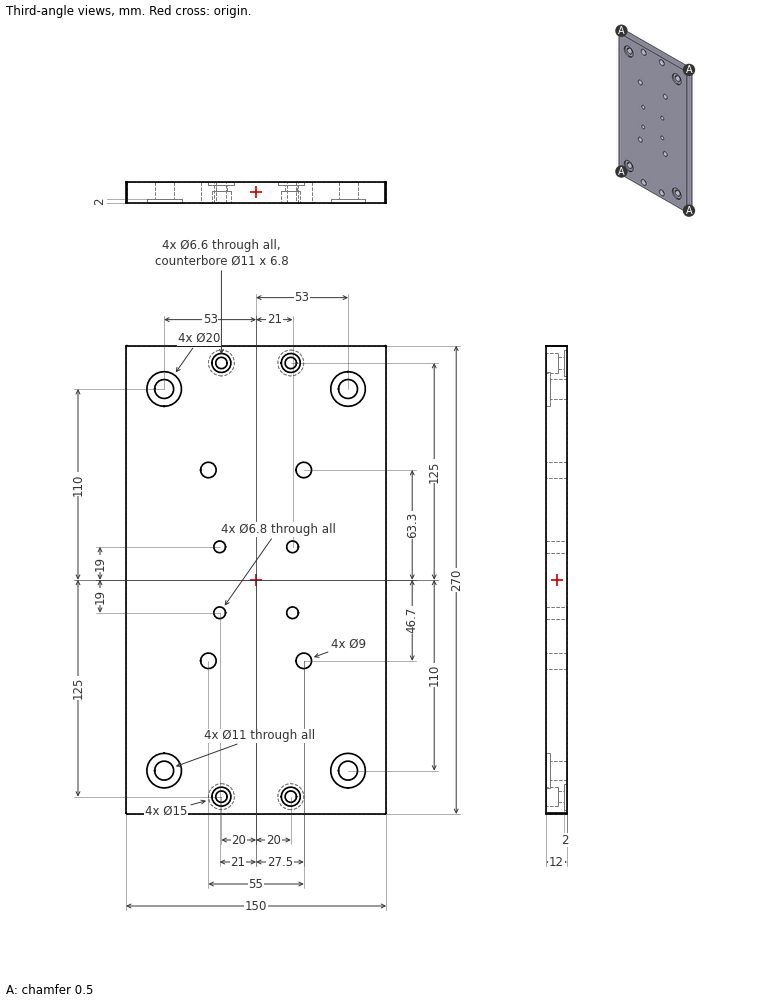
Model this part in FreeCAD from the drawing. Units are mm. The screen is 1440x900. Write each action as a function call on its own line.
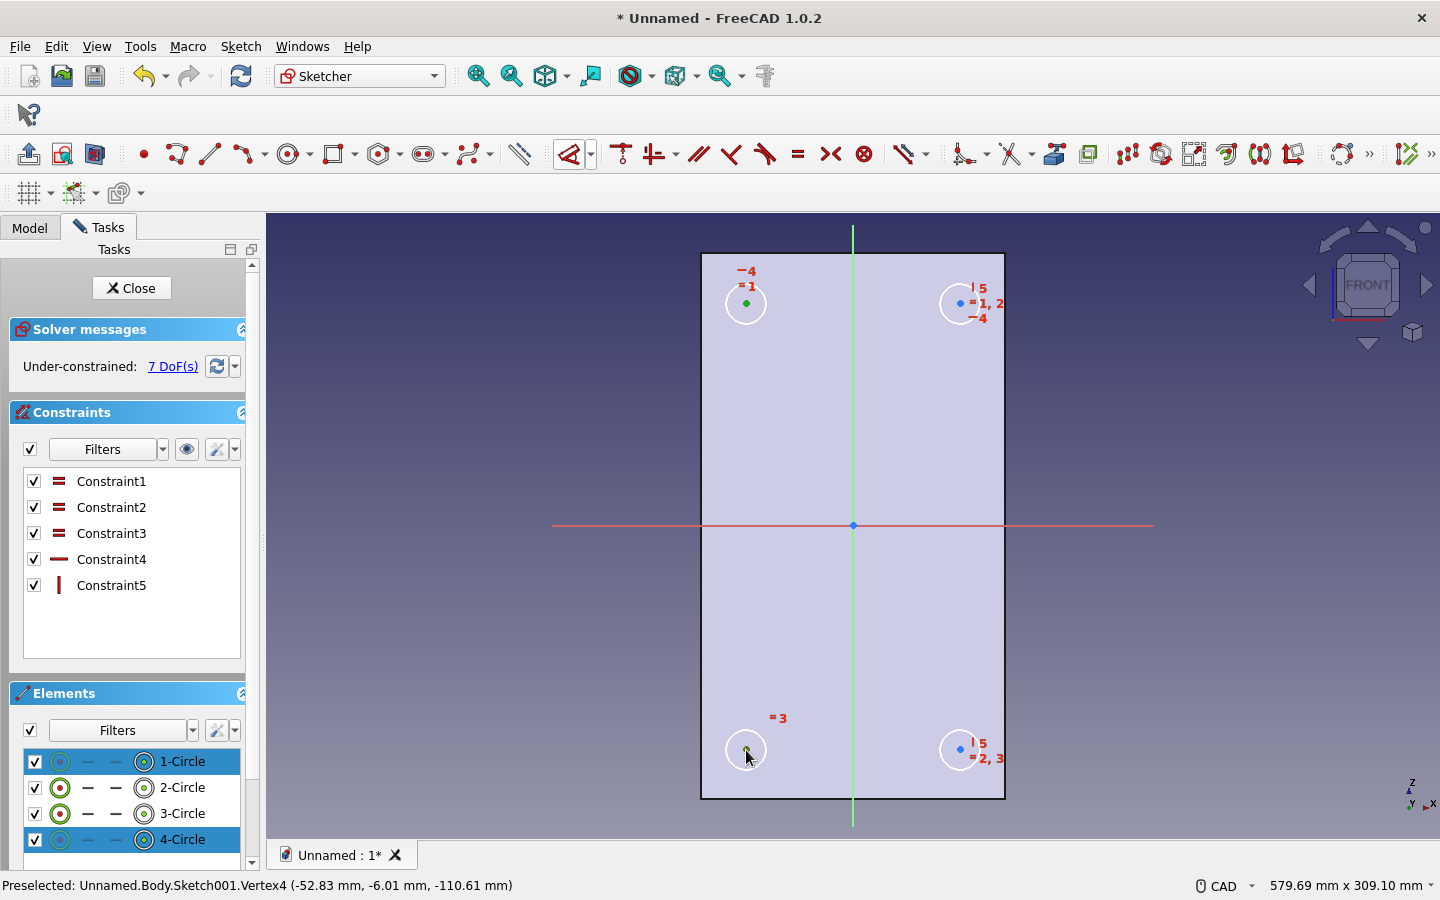
key(v)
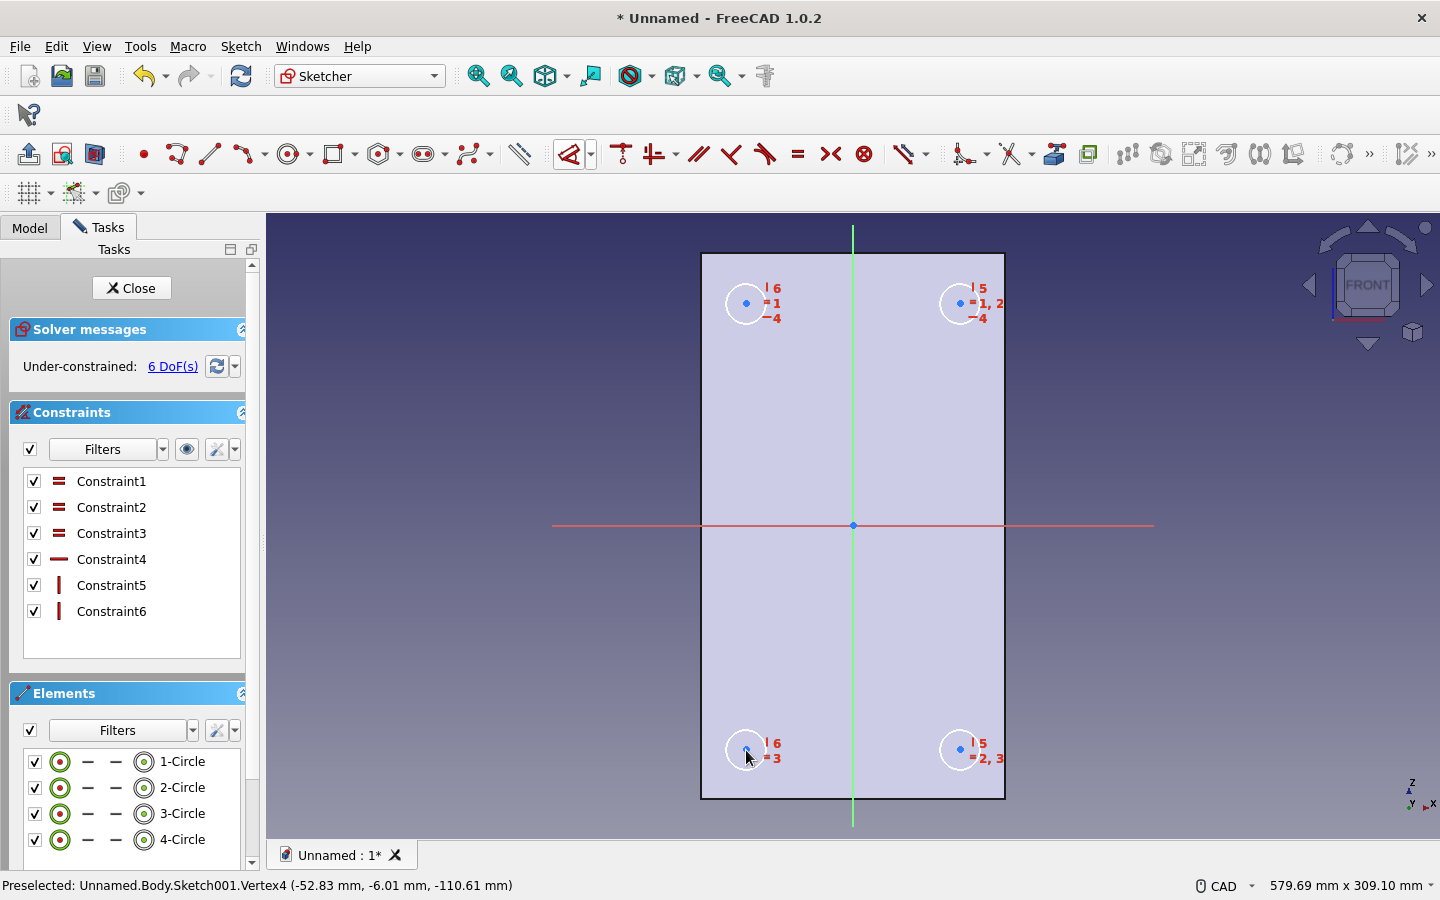
click(960, 750)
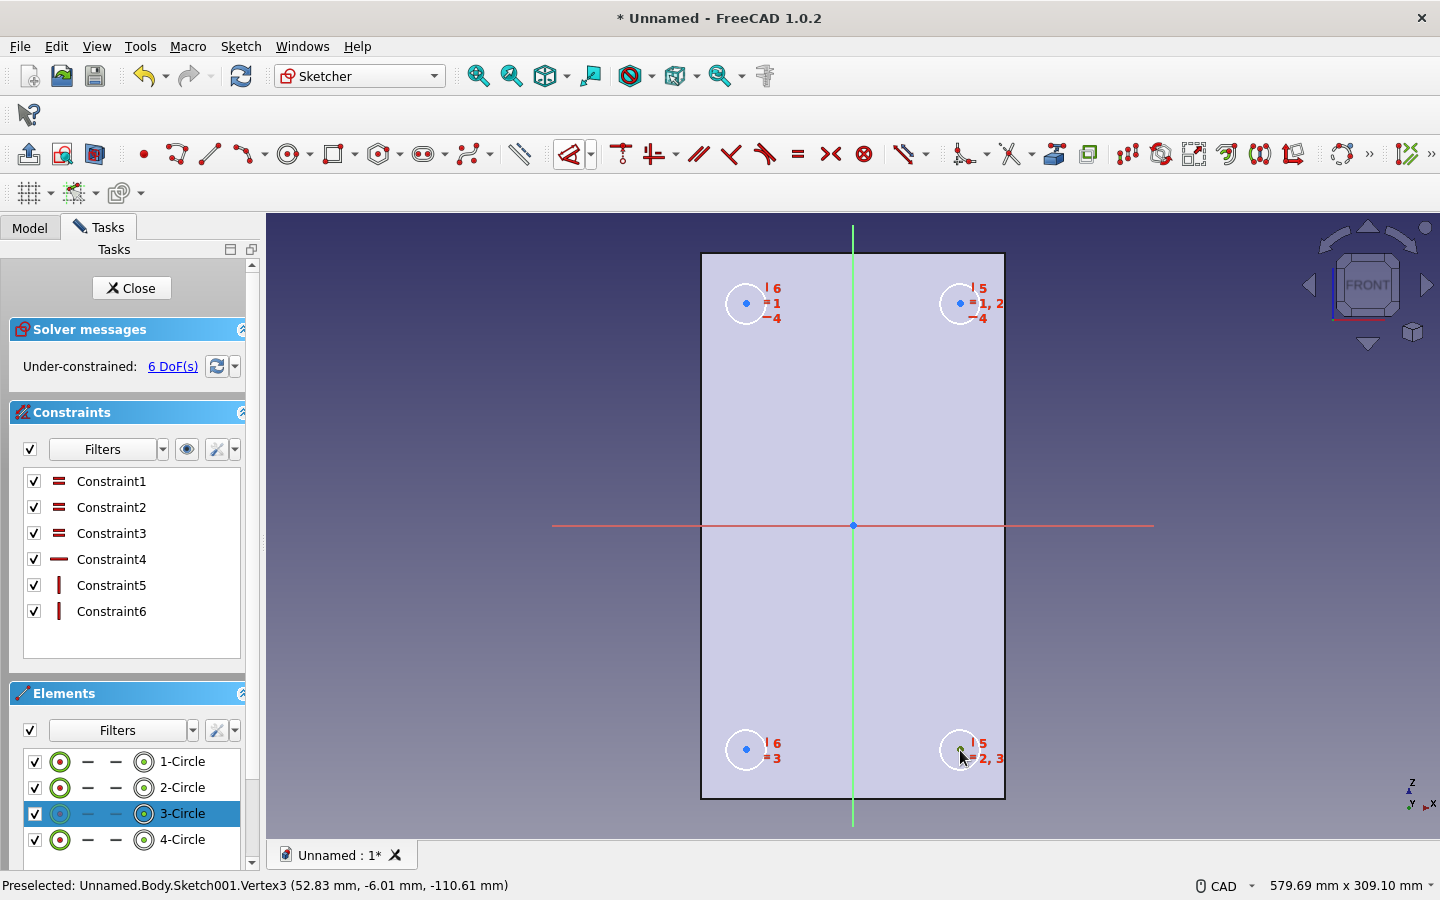
click(746, 750)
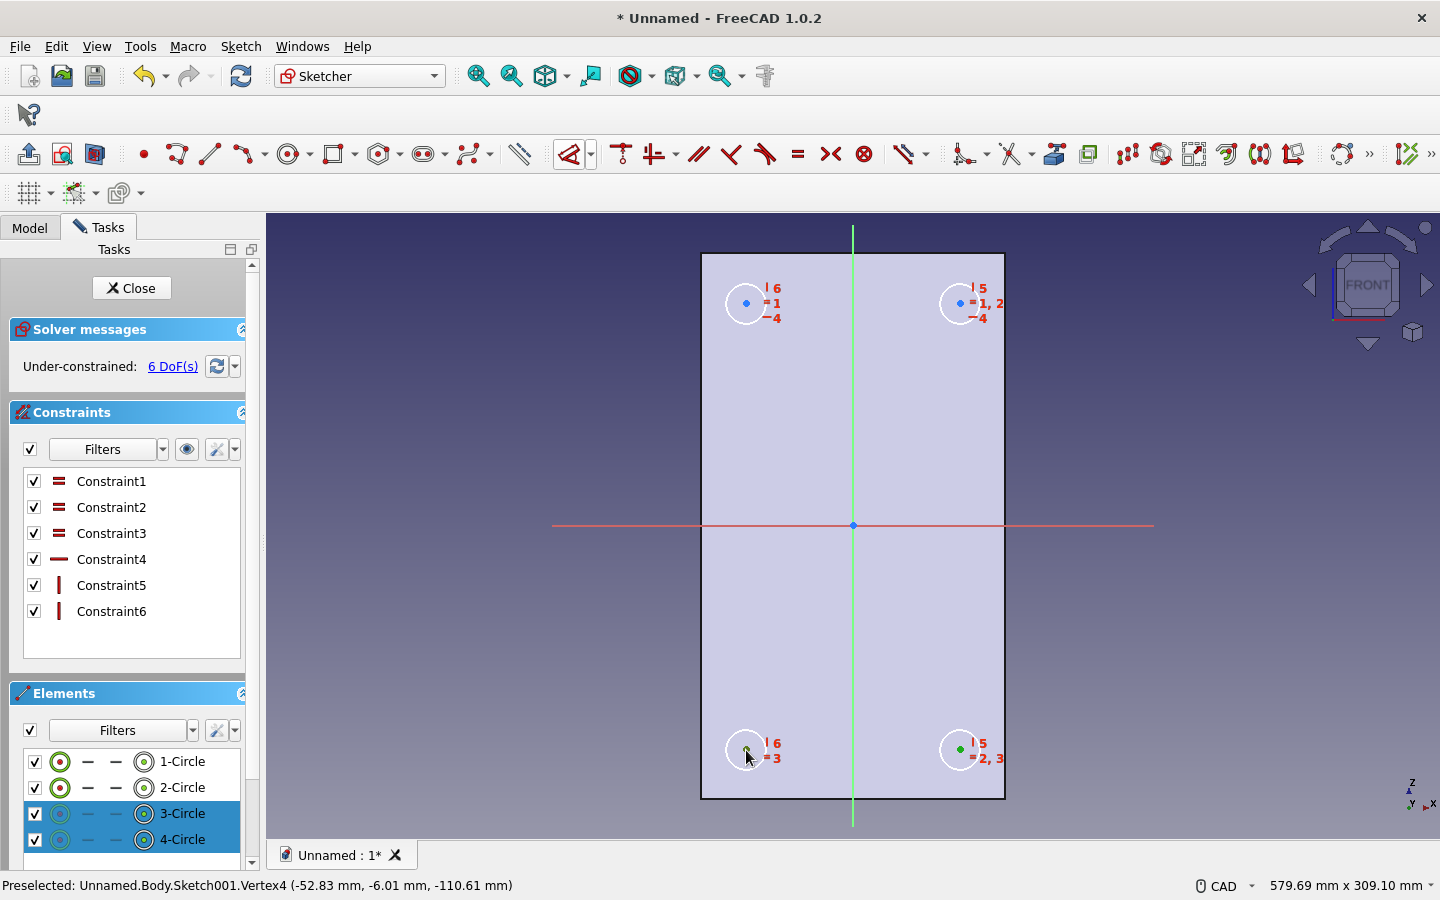
key(h)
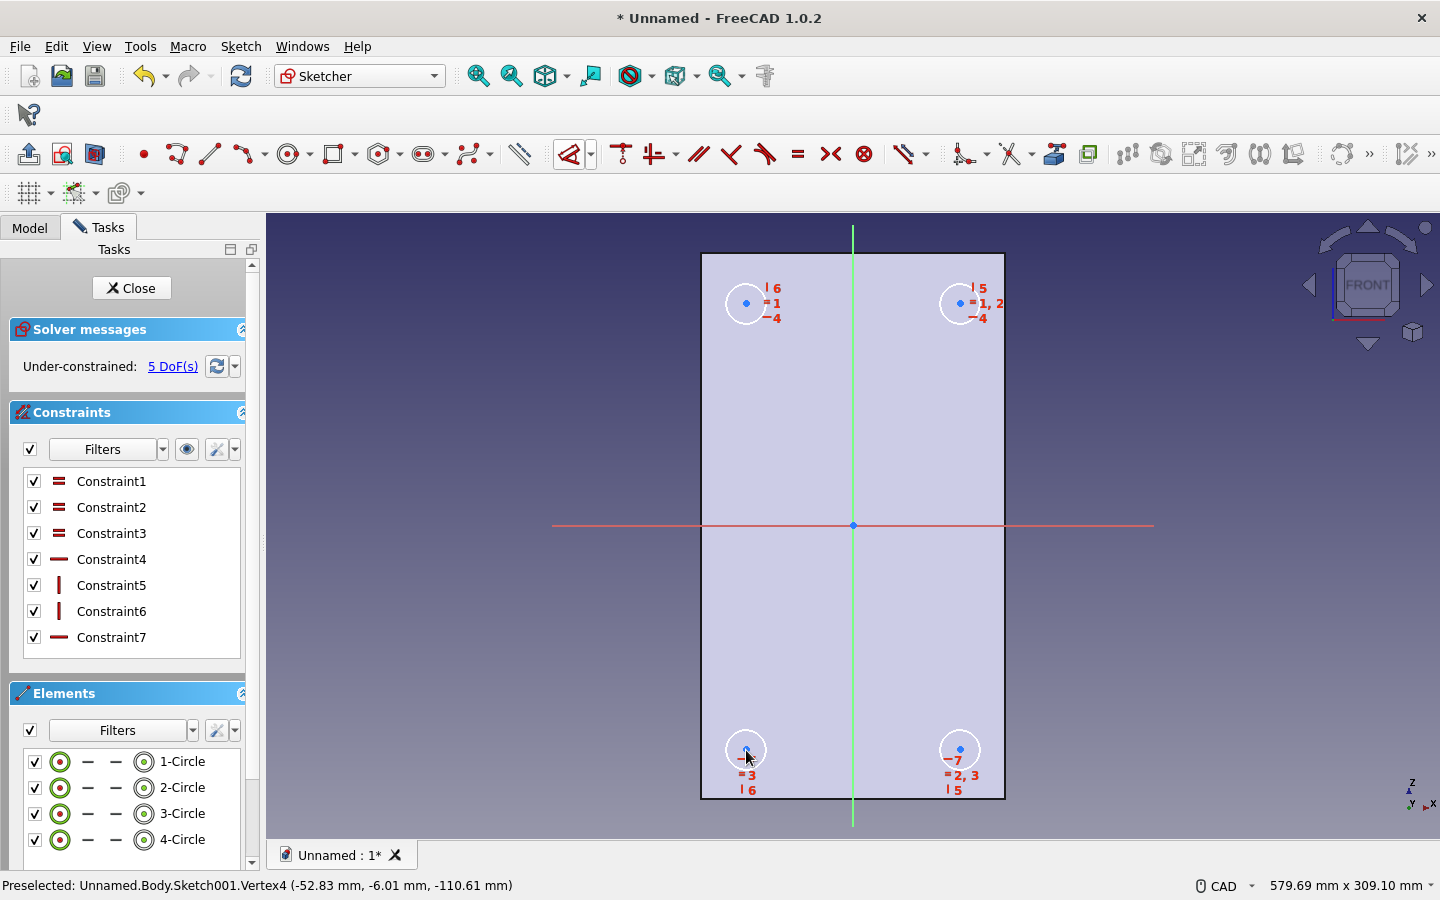
click(760, 290)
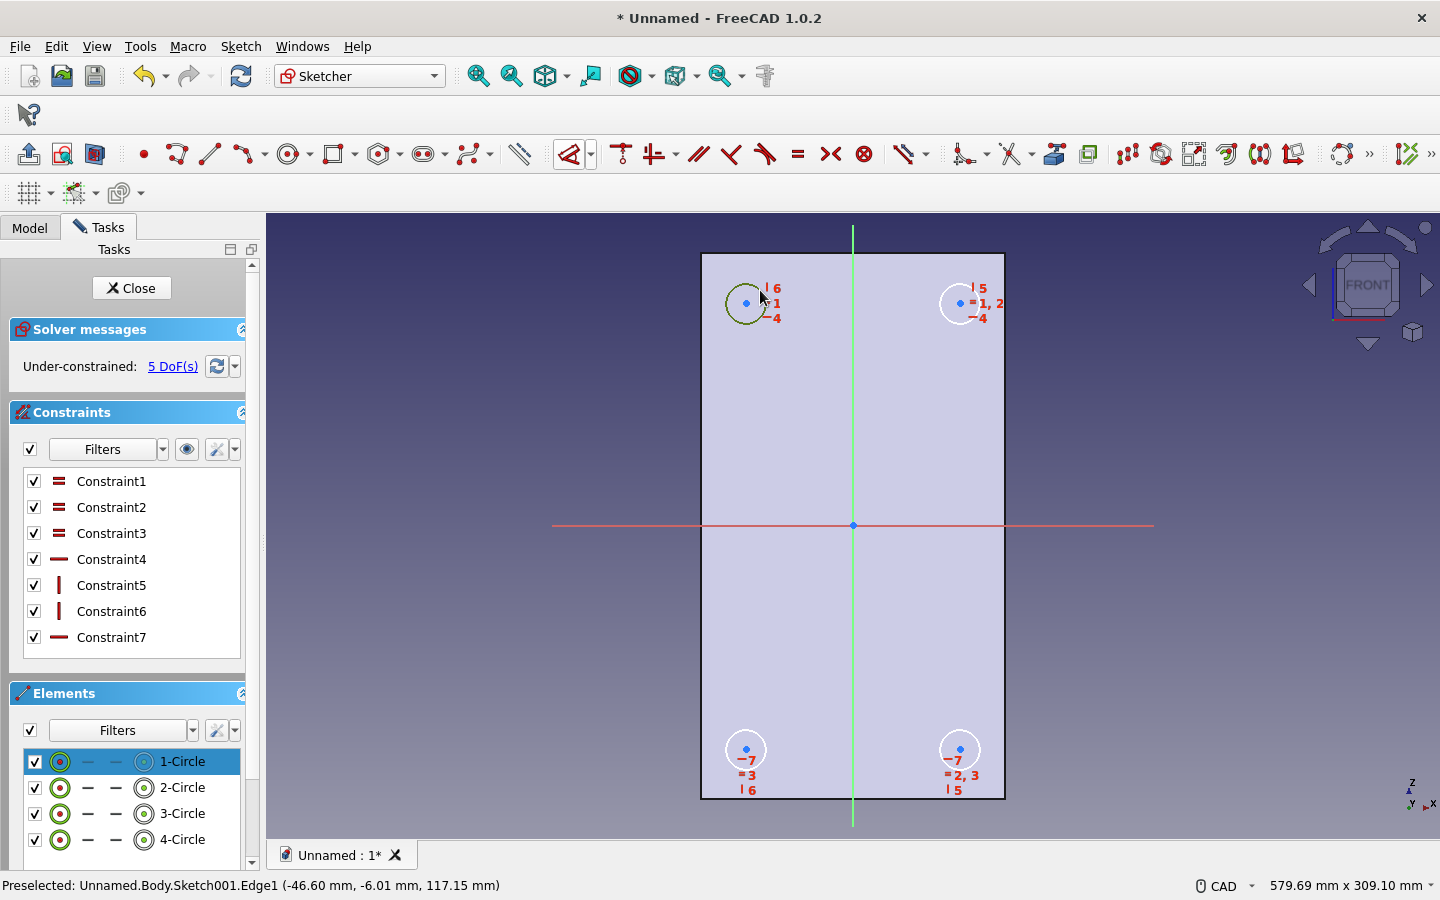
click(590, 154)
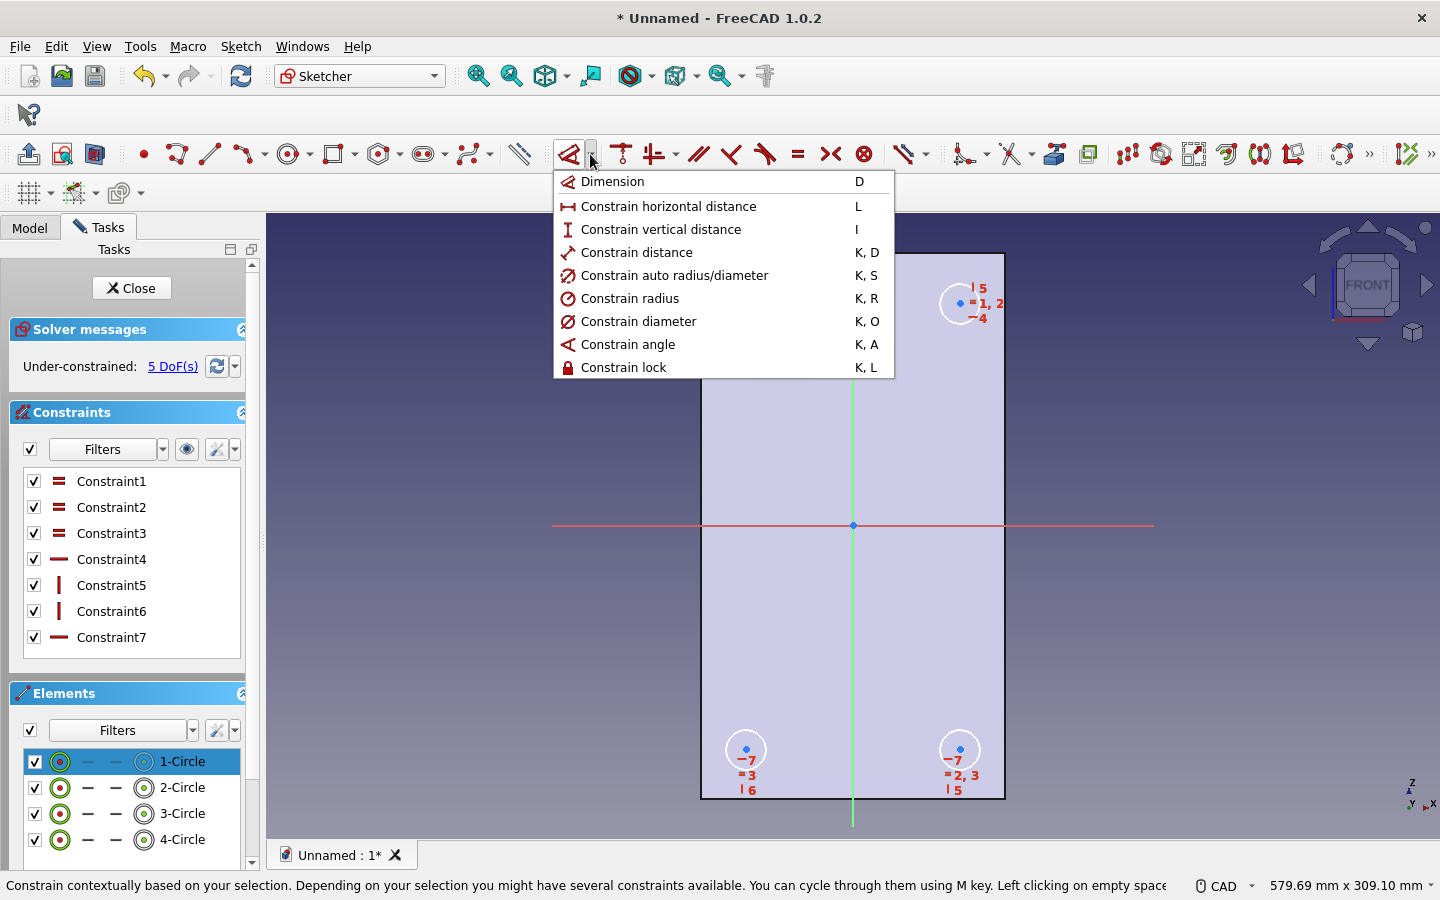
click(724, 322)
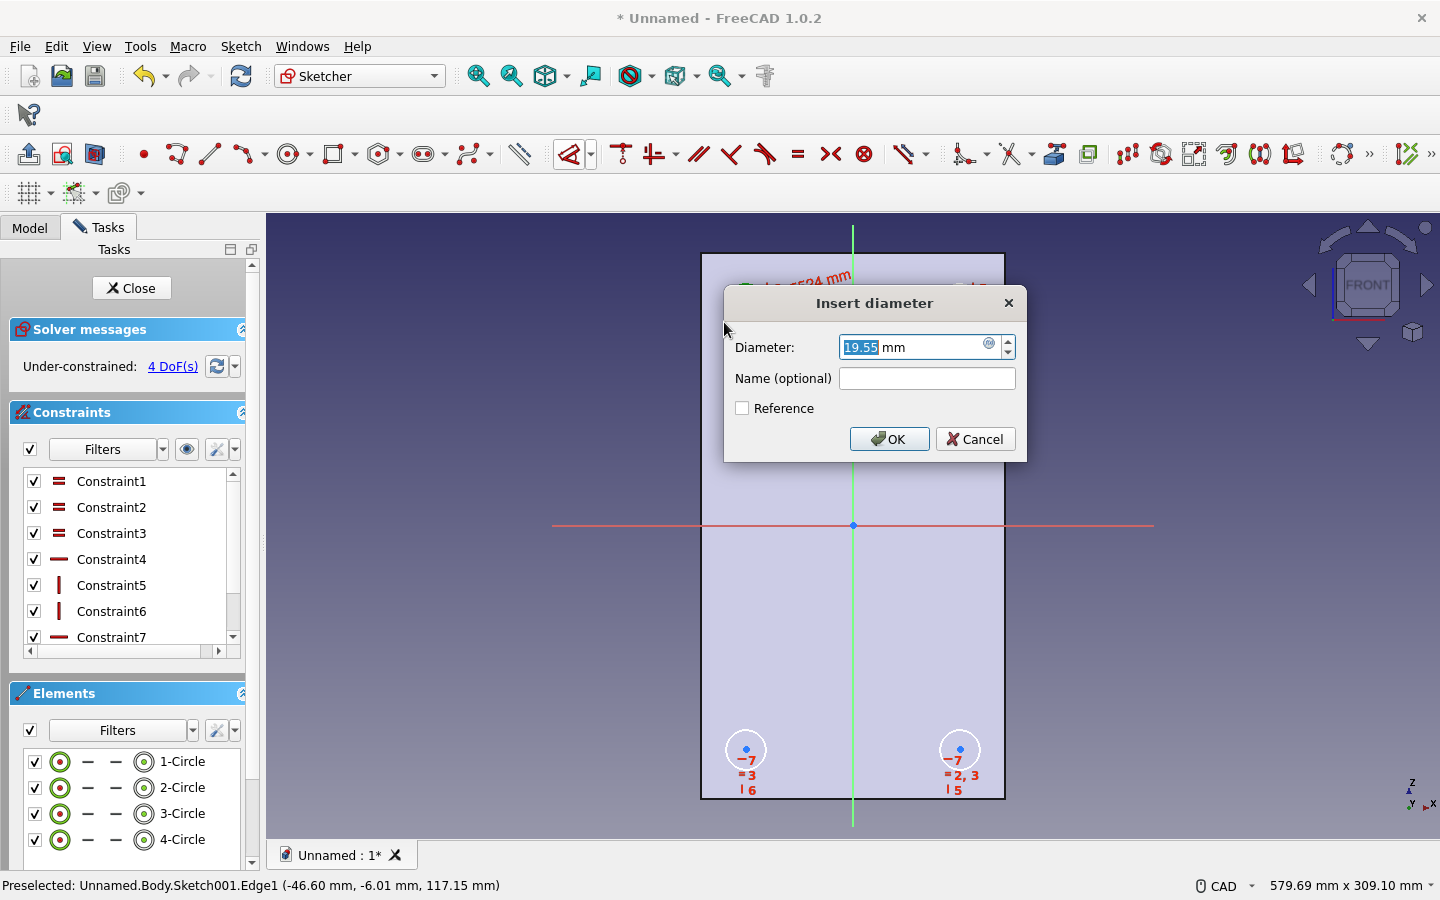
text(20)
key(Return)